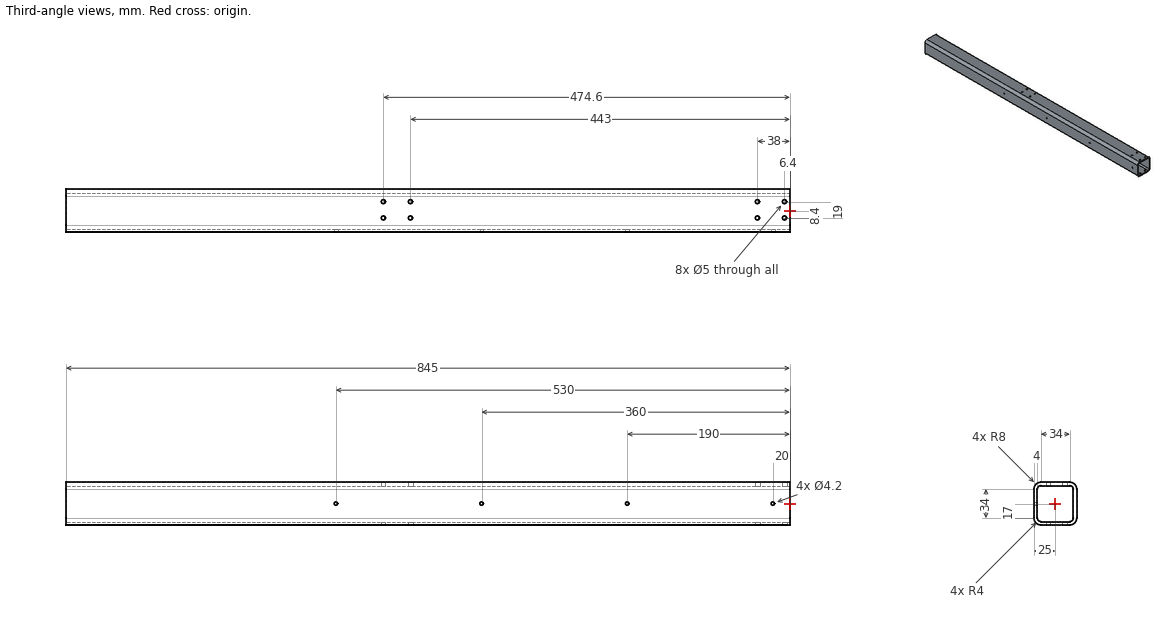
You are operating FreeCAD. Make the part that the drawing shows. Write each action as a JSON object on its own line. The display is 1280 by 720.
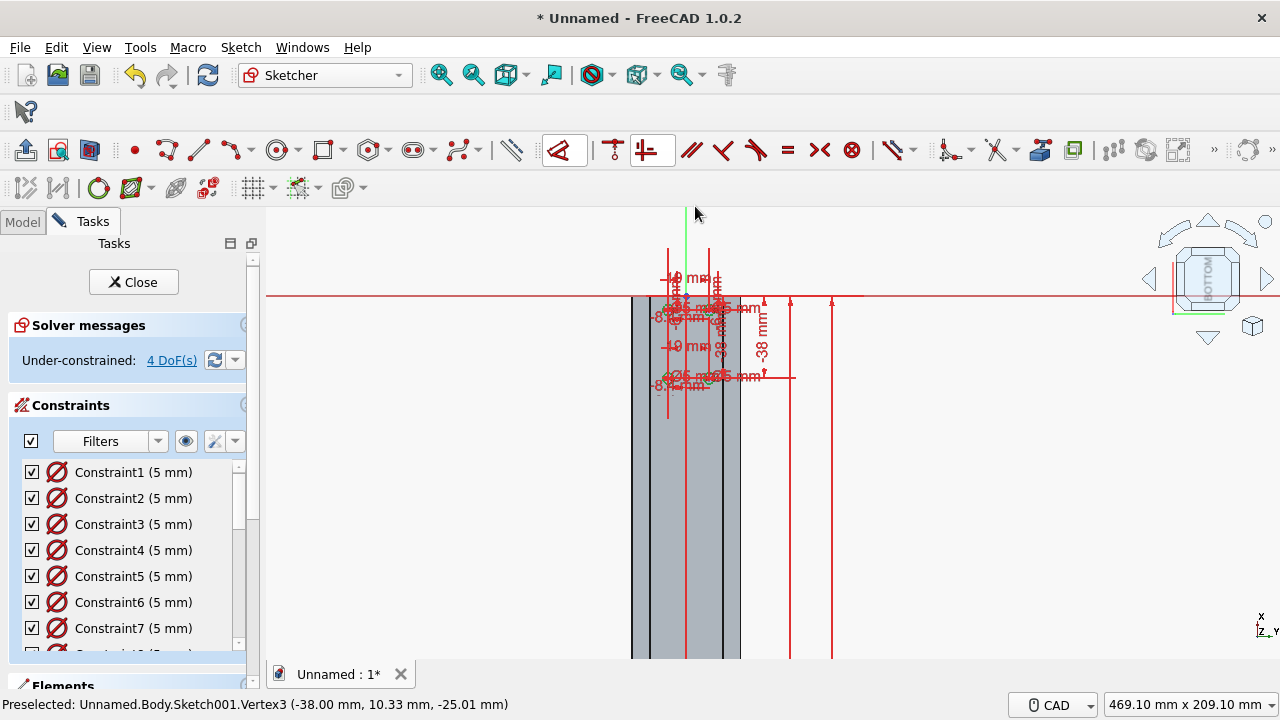
{"action": "left_click", "coordinate": [668, 378]}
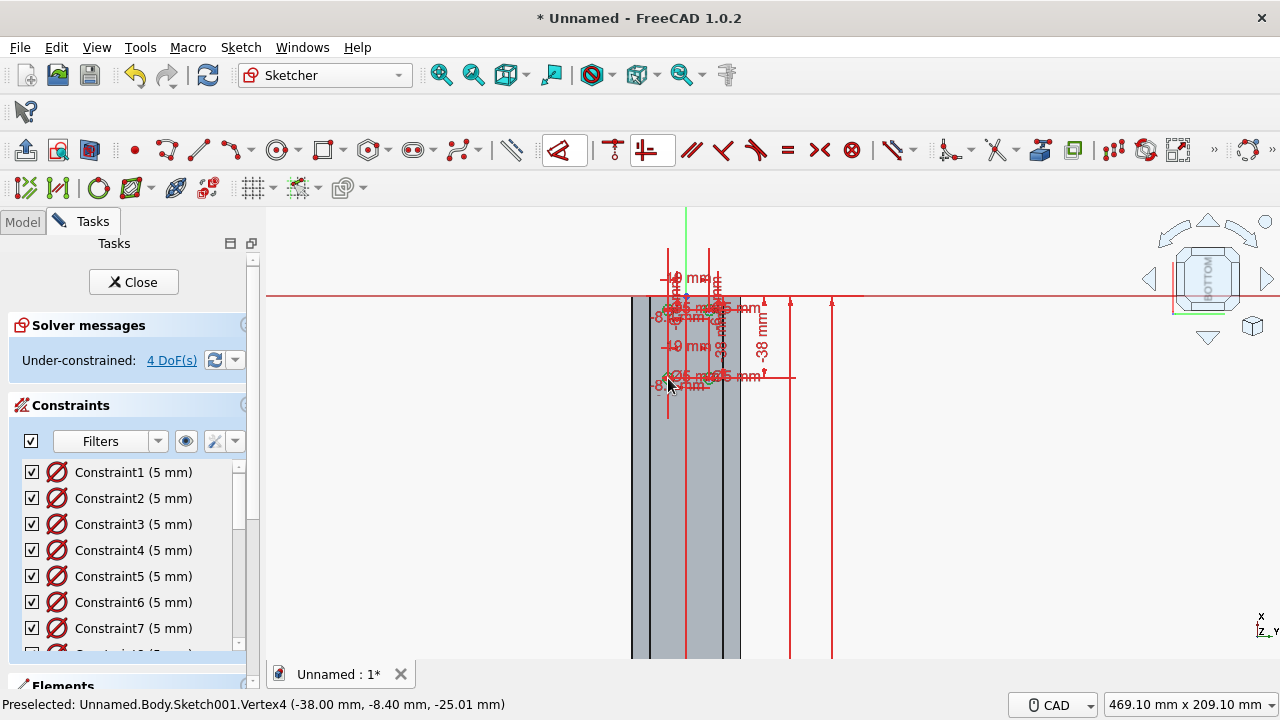
{"action": "scroll", "coordinate": [710, 309], "scroll_direction": "down", "scroll_amount": 7}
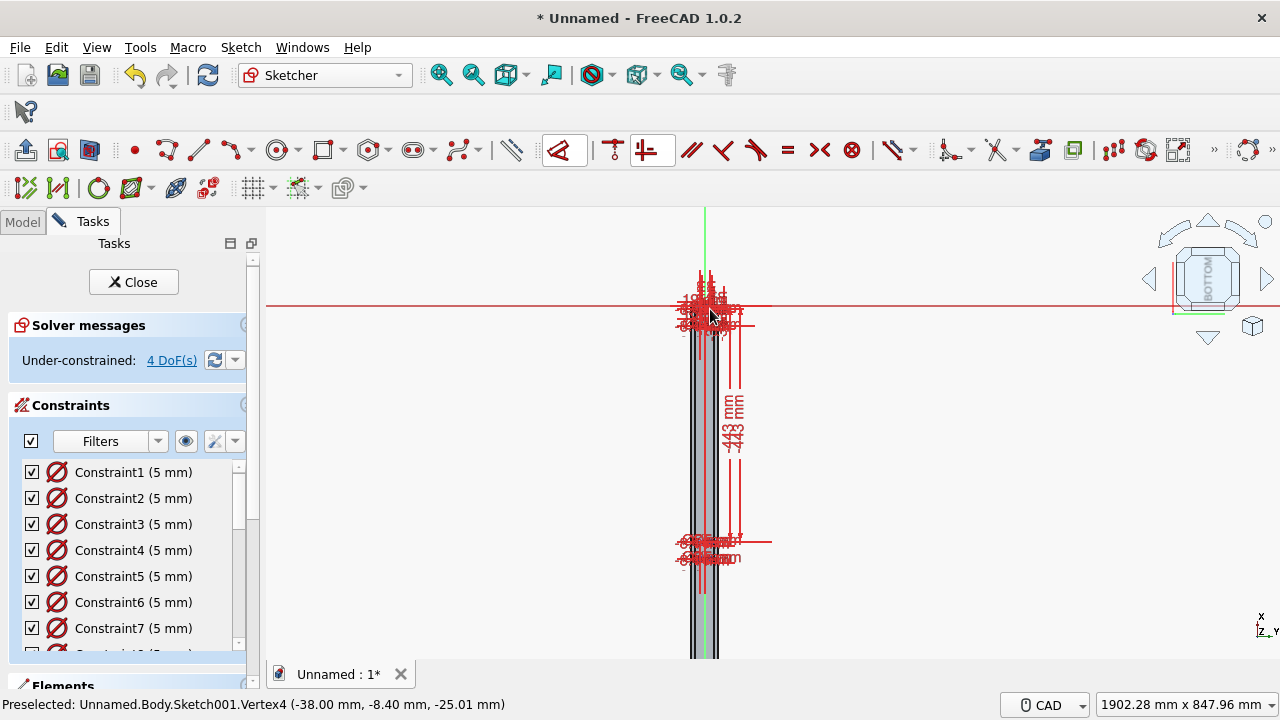
{"action": "scroll", "coordinate": [710, 542], "scroll_direction": "up", "scroll_amount": 7}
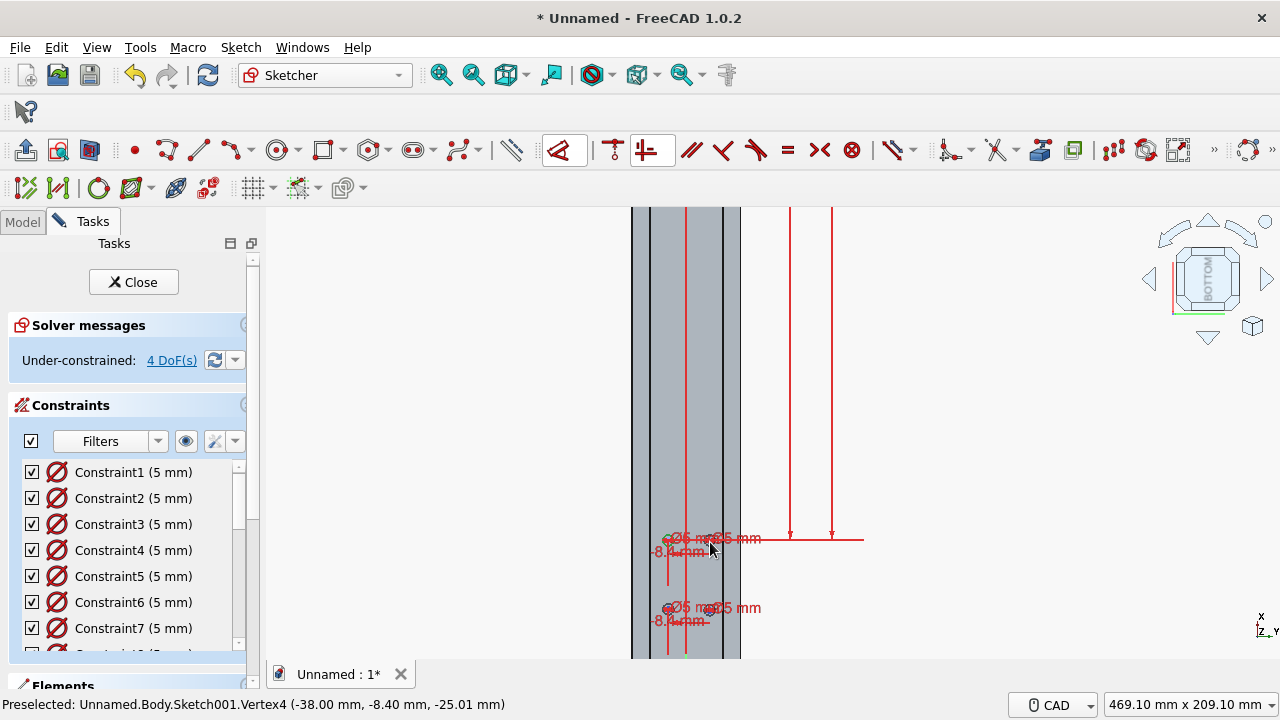
{"action": "left_click", "coordinate": [710, 540]}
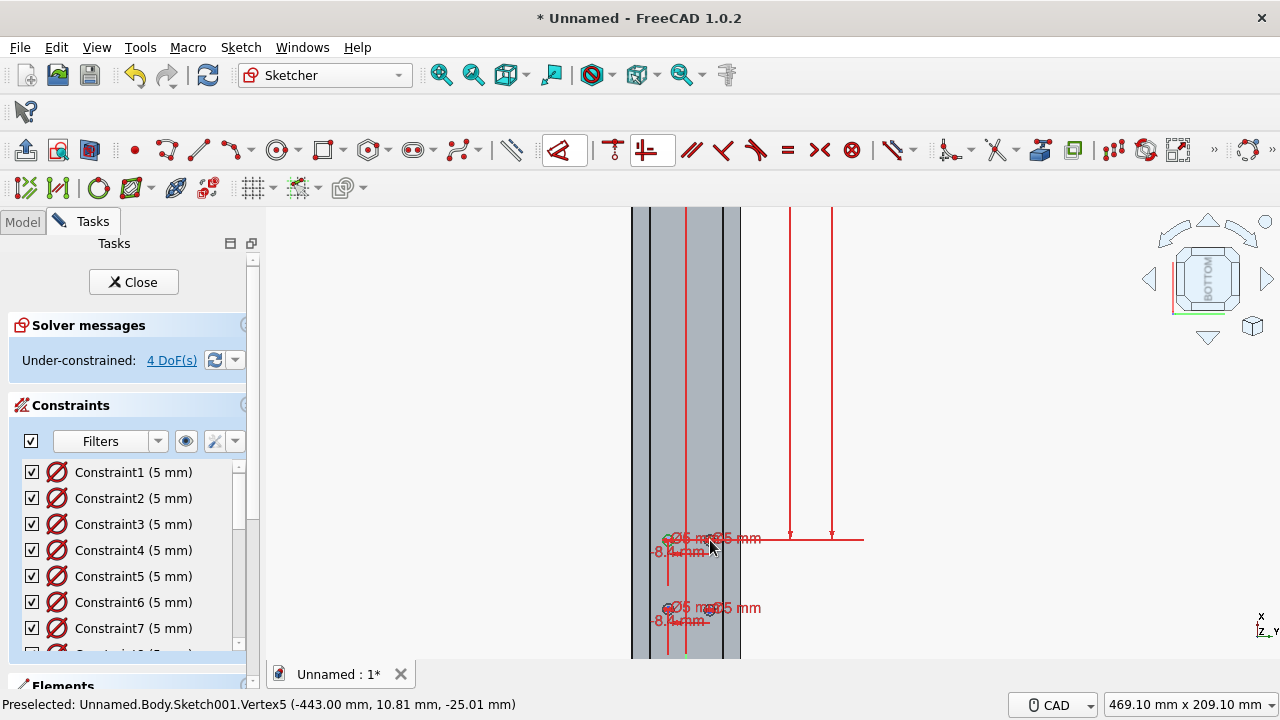
{"action": "key", "text": "l"}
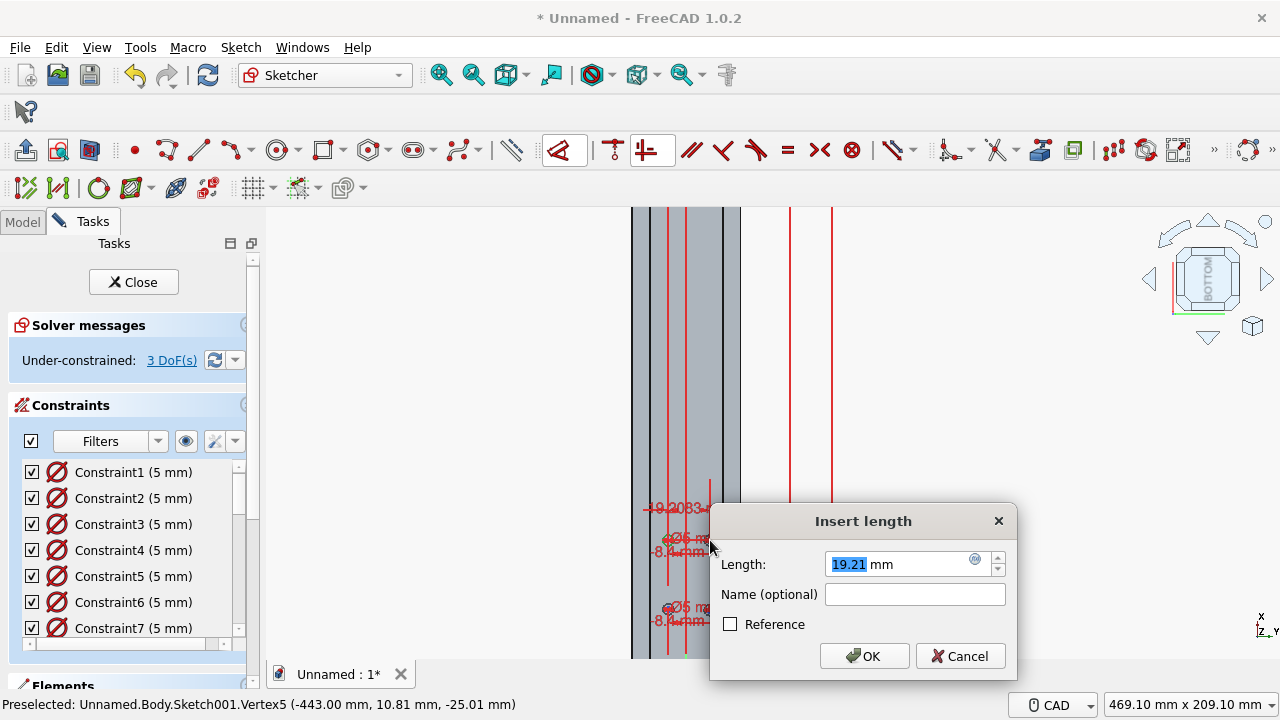
{"action": "type", "text": "19"}
{"action": "key", "text": "Return"}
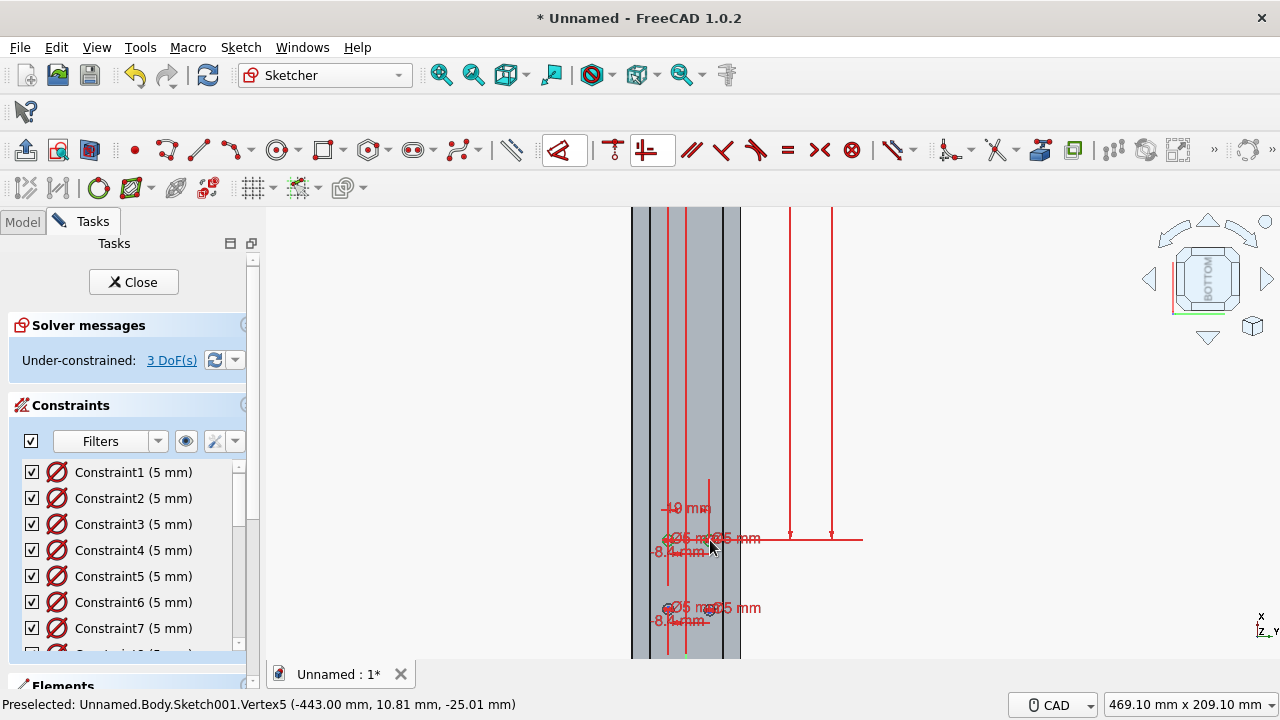
{"action": "left_click", "coordinate": [668, 540]}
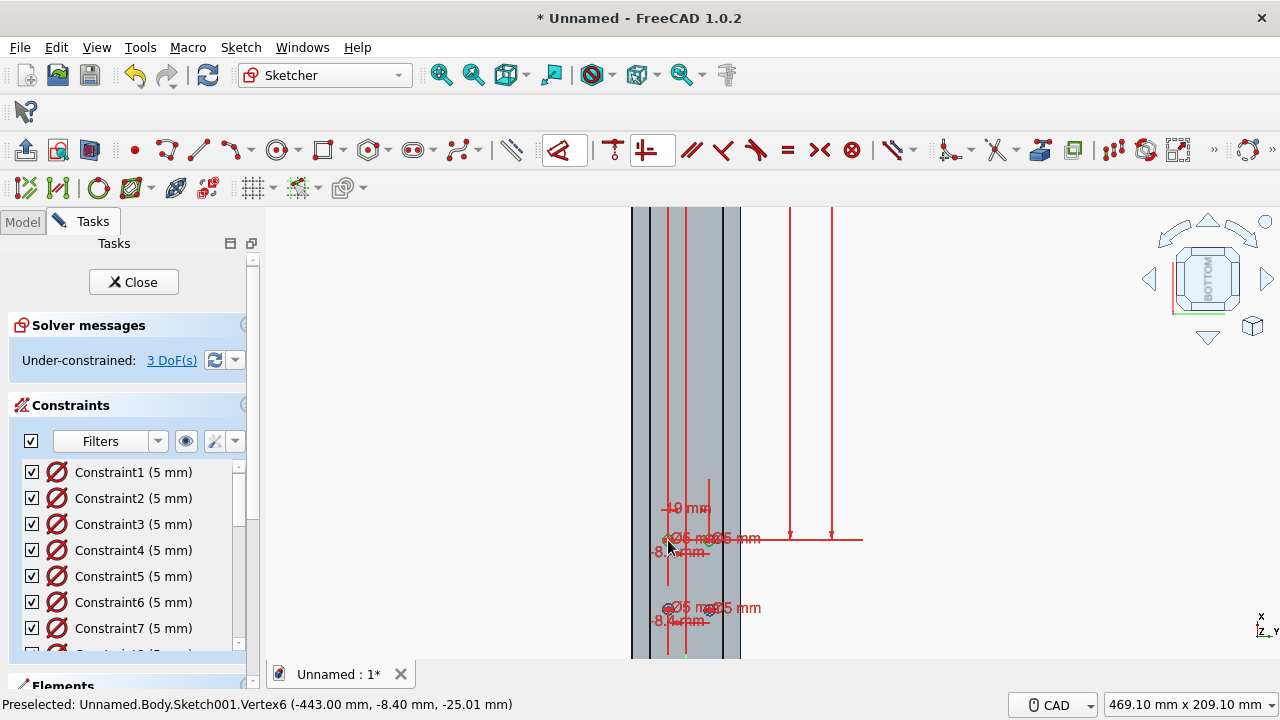
{"action": "left_click", "coordinate": [710, 610]}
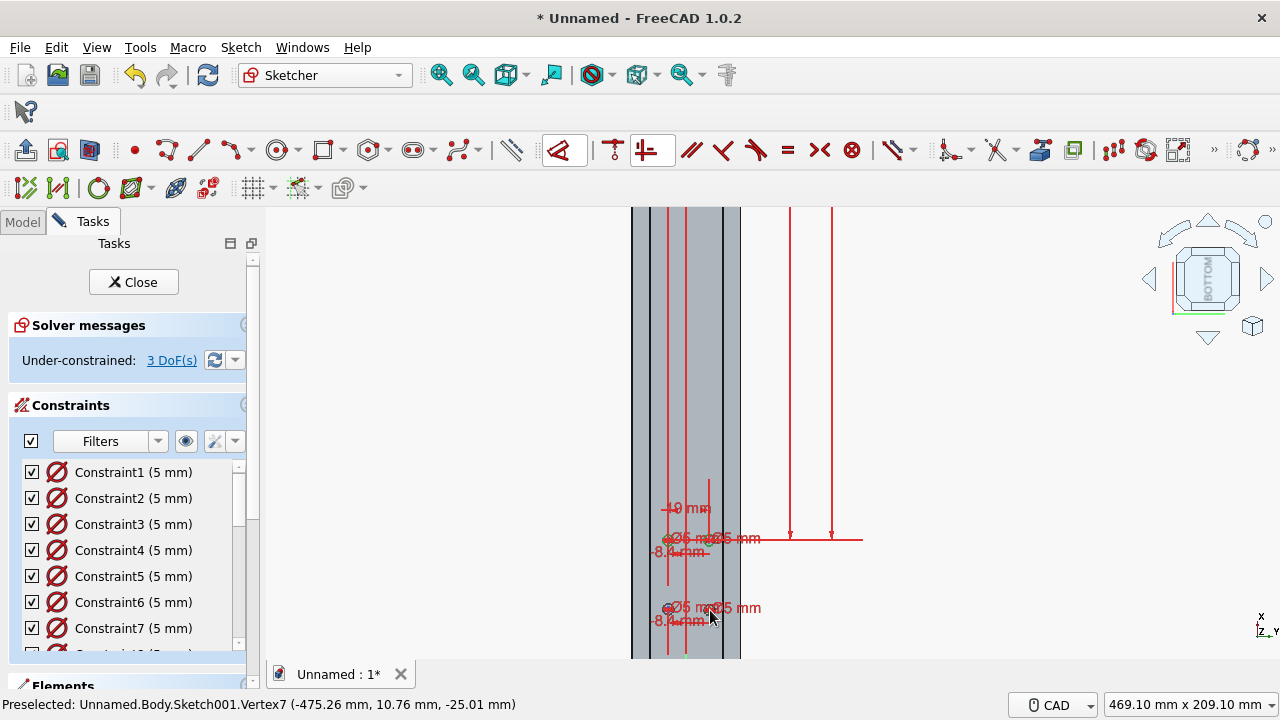
{"action": "left_click", "coordinate": [582, 150]}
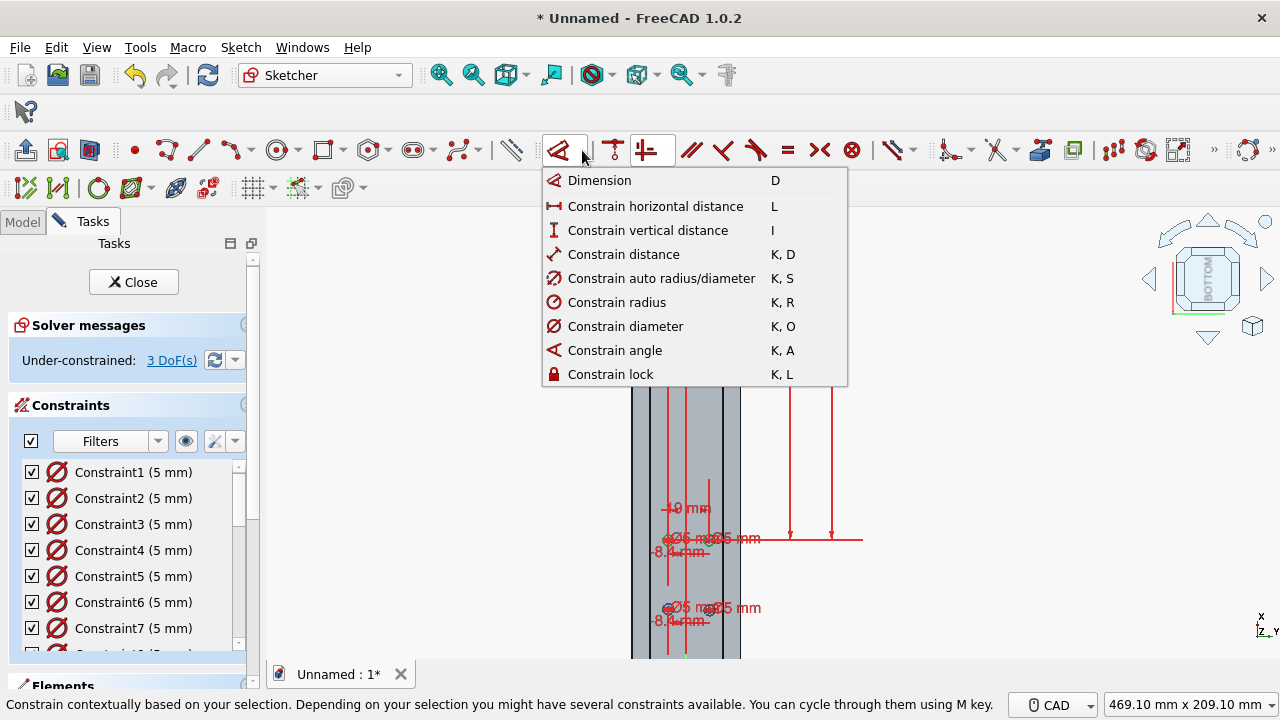
{"action": "left_click", "coordinate": [695, 206]}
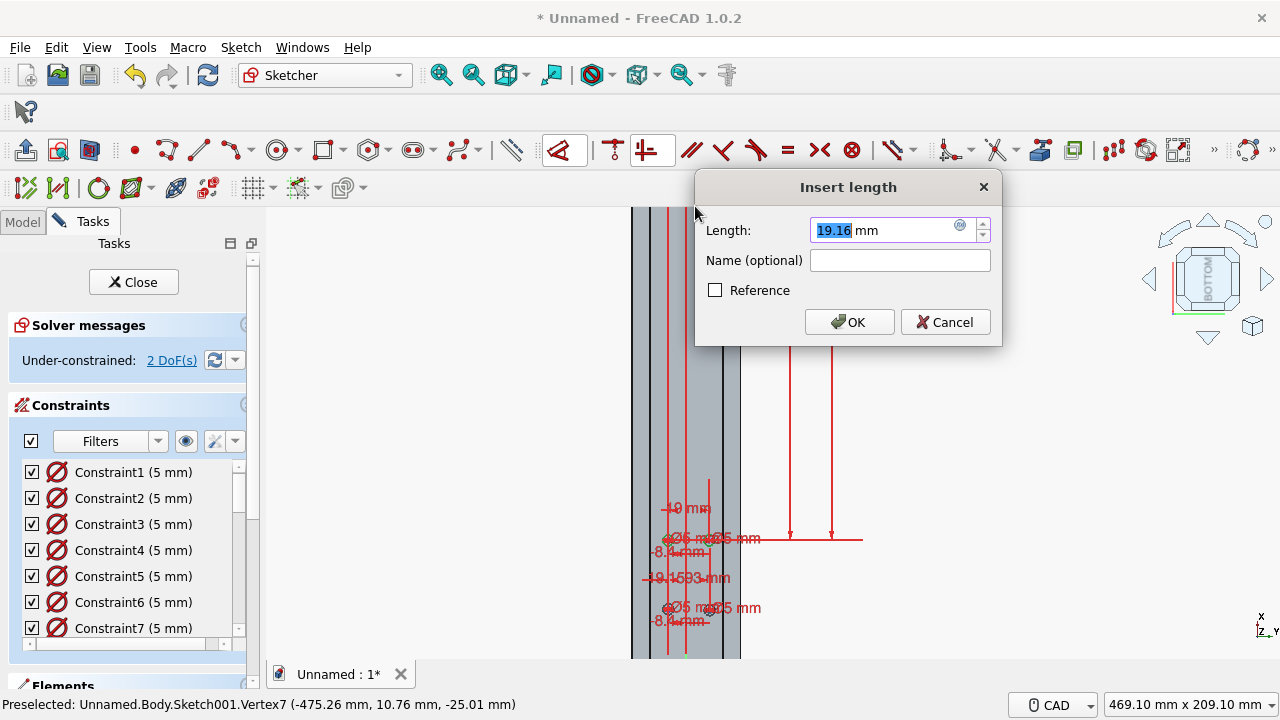
{"action": "type", "text": "19"}
{"action": "key", "text": "Return"}